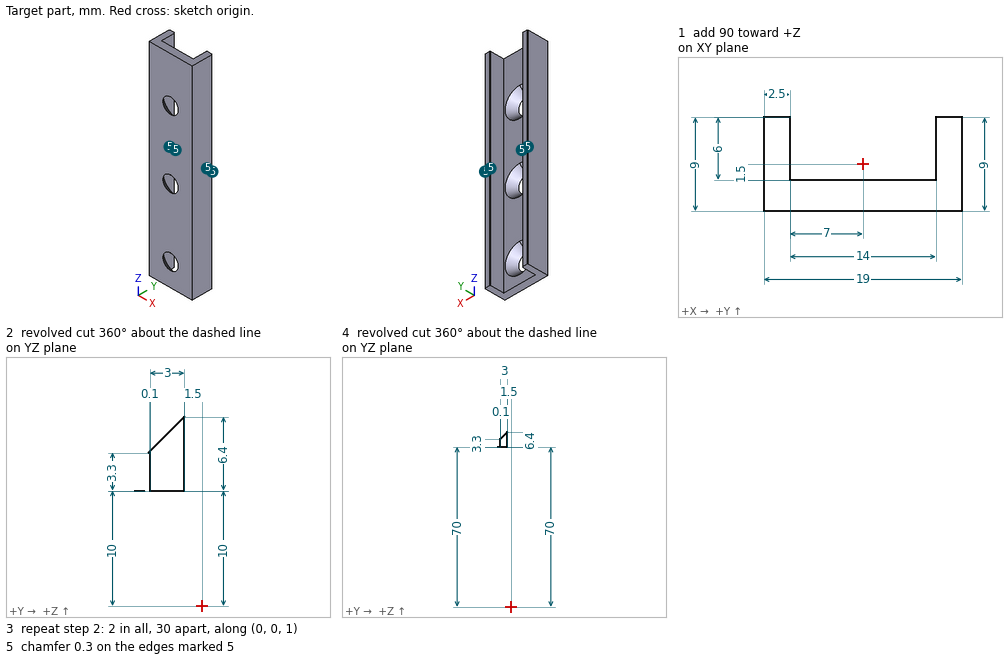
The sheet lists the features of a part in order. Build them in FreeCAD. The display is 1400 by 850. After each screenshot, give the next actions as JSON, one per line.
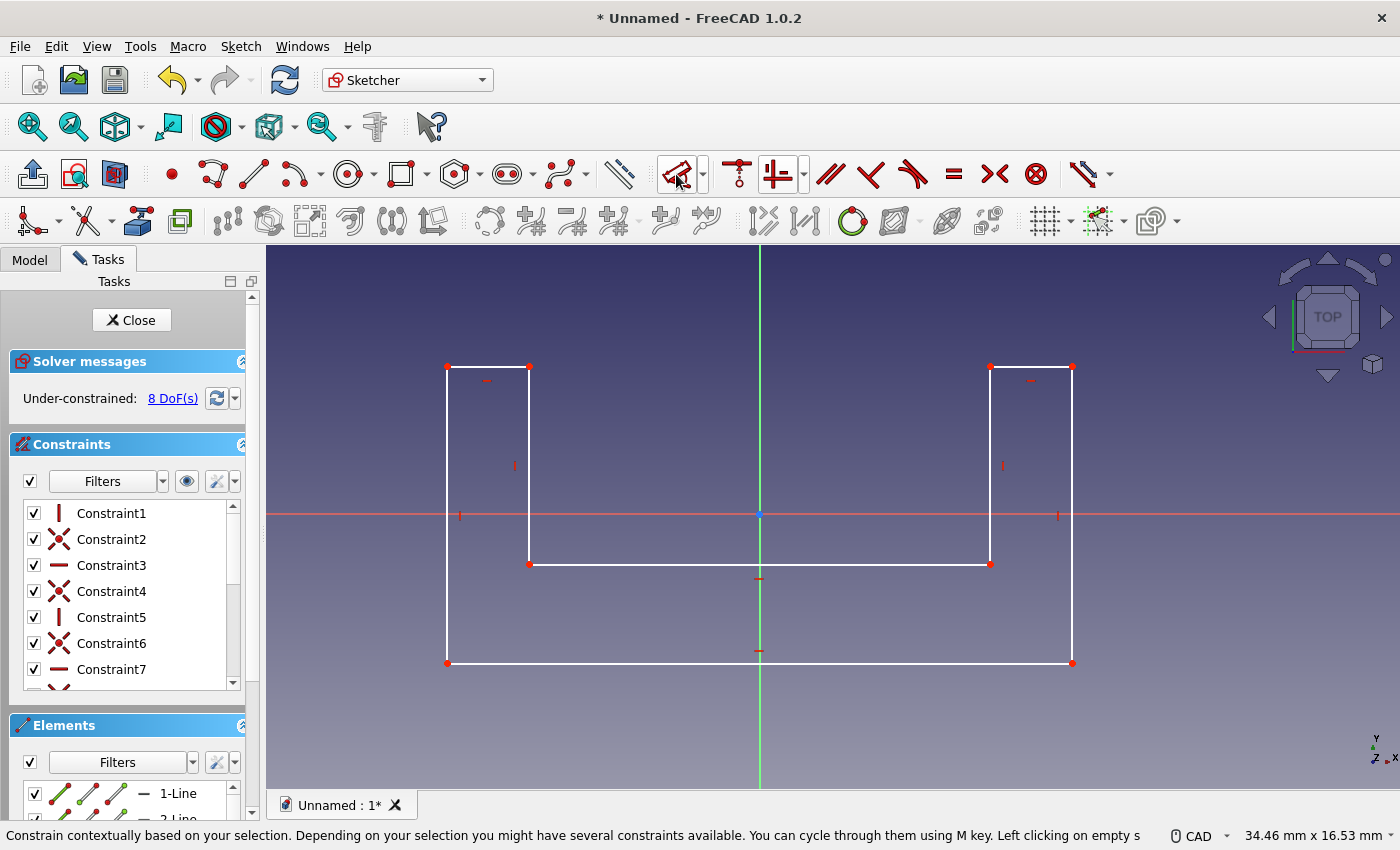
{"action": "left_click", "coordinate": [529, 426]}
{"action": "left_click", "coordinate": [495, 466]}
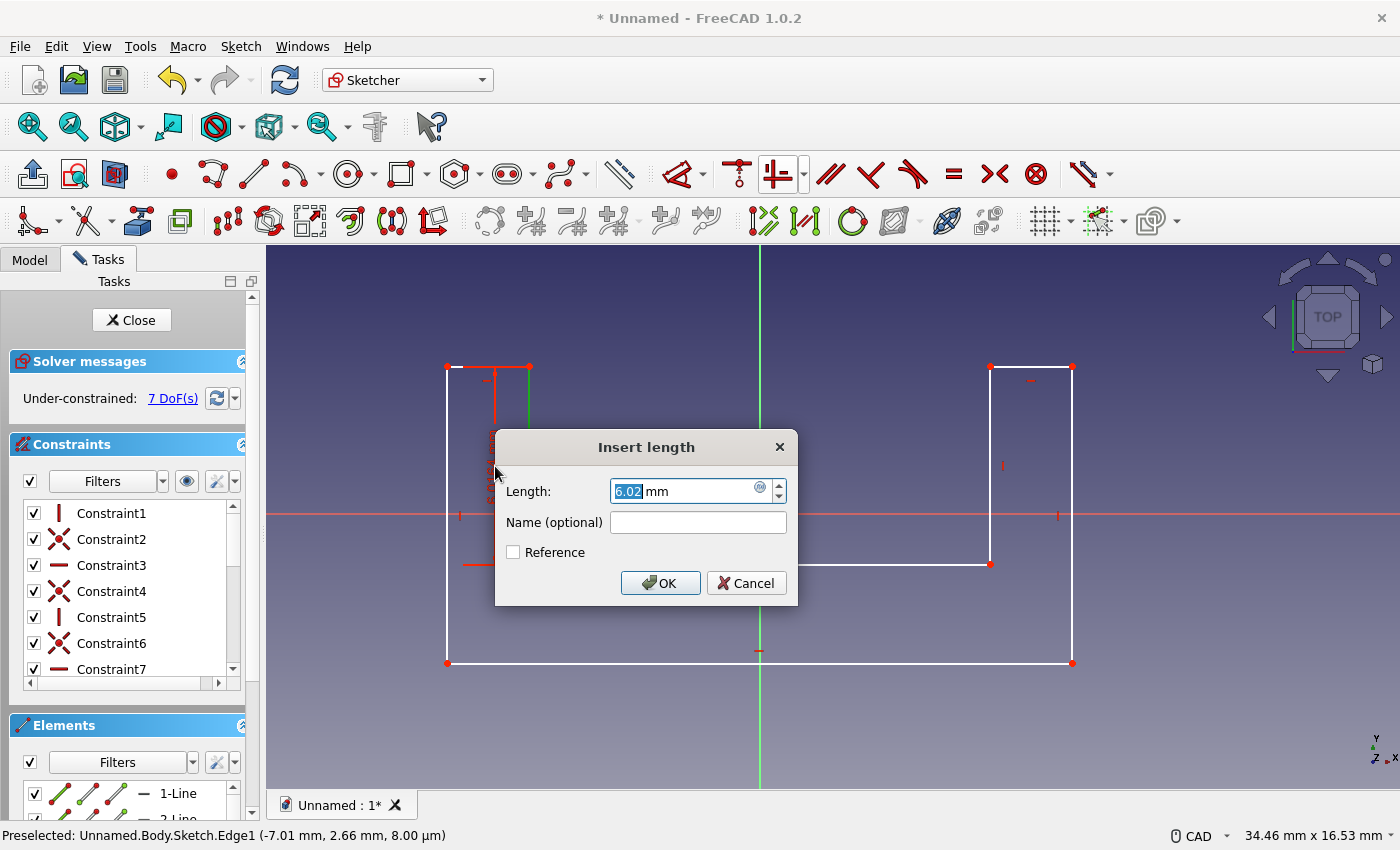
{"action": "type", "text": "6"}
{"action": "key", "text": "Return"}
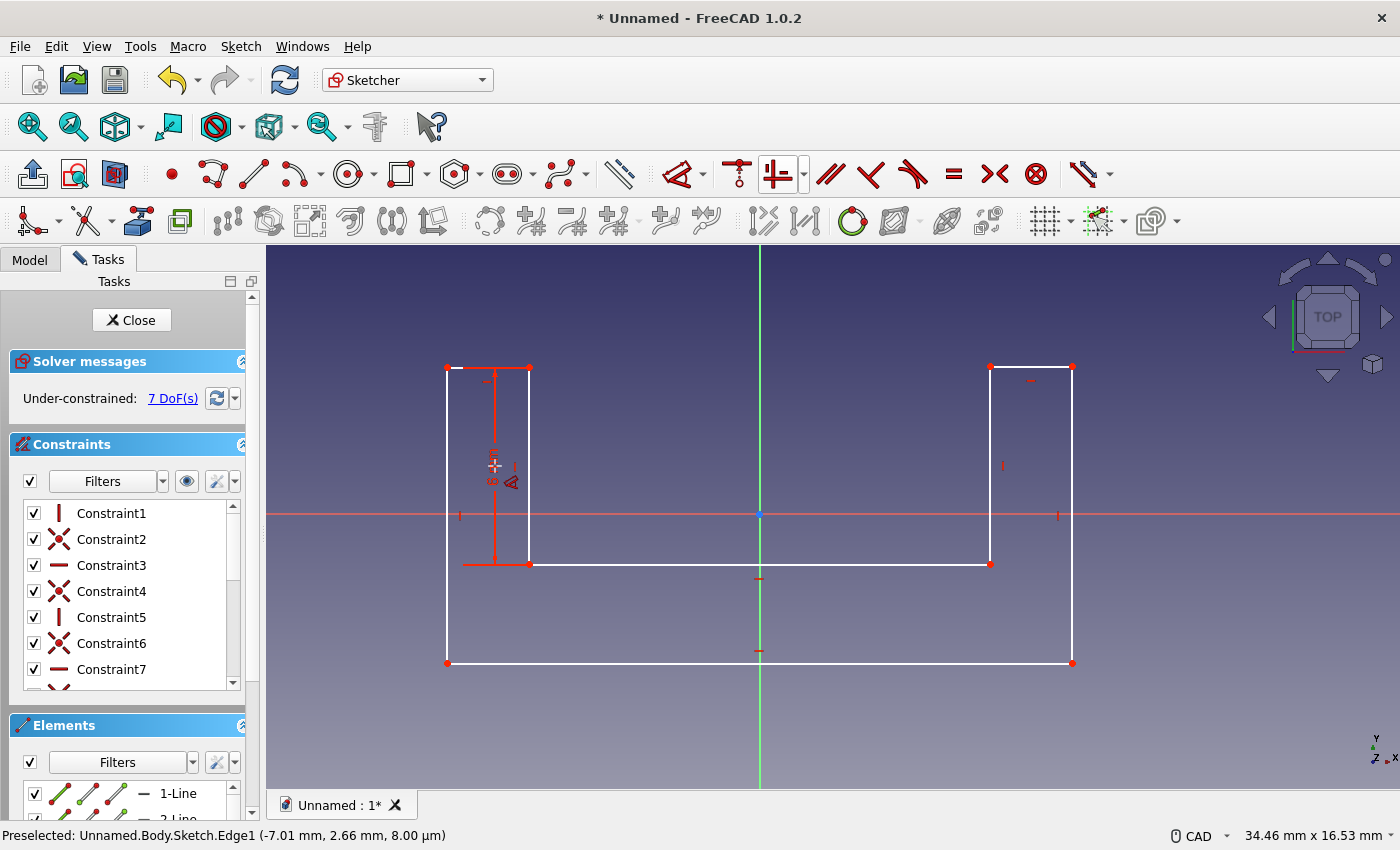
{"action": "left_click", "coordinate": [447, 456]}
{"action": "left_click", "coordinate": [413, 448]}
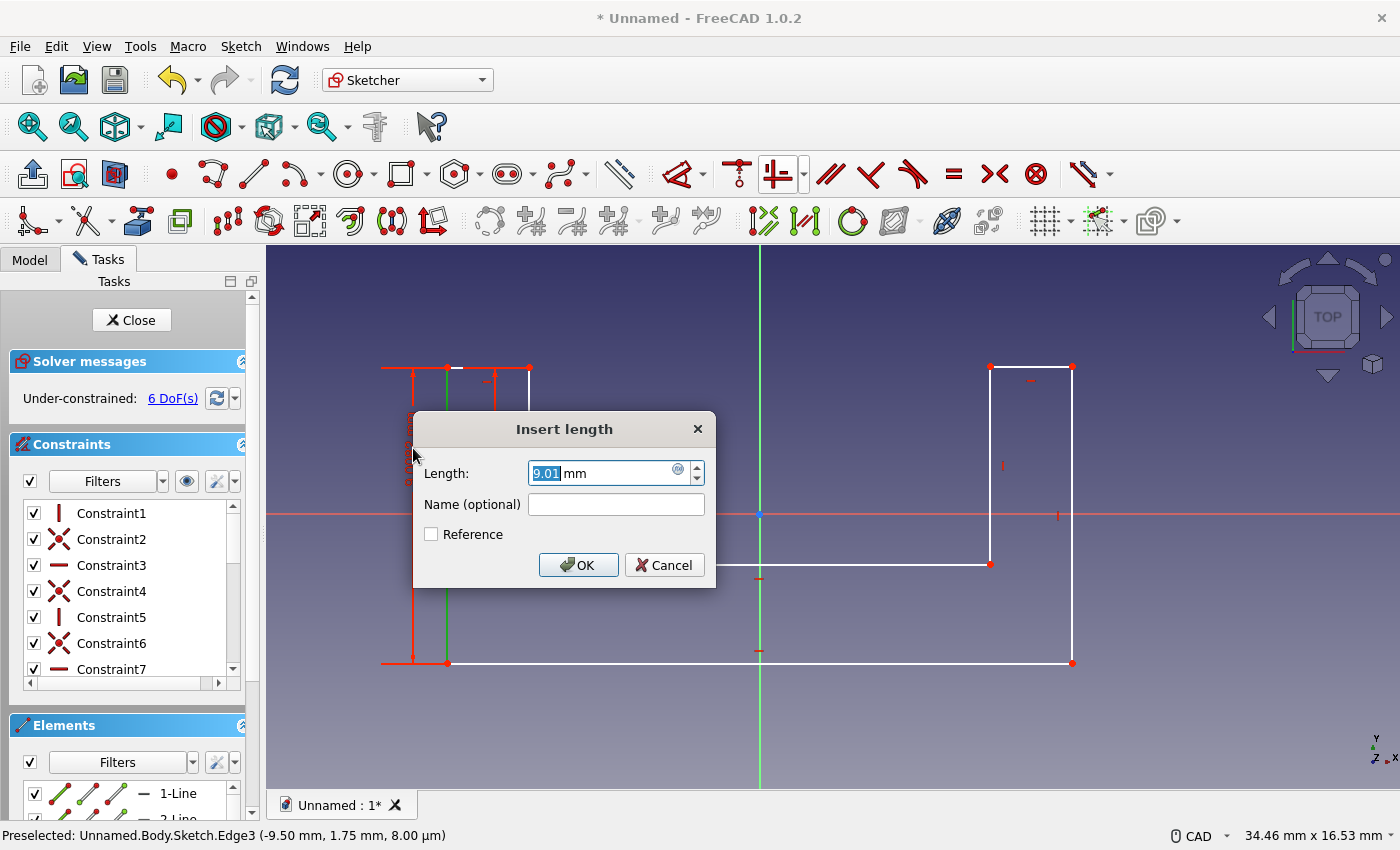
{"action": "type", "text": "9"}
{"action": "key", "text": "Return"}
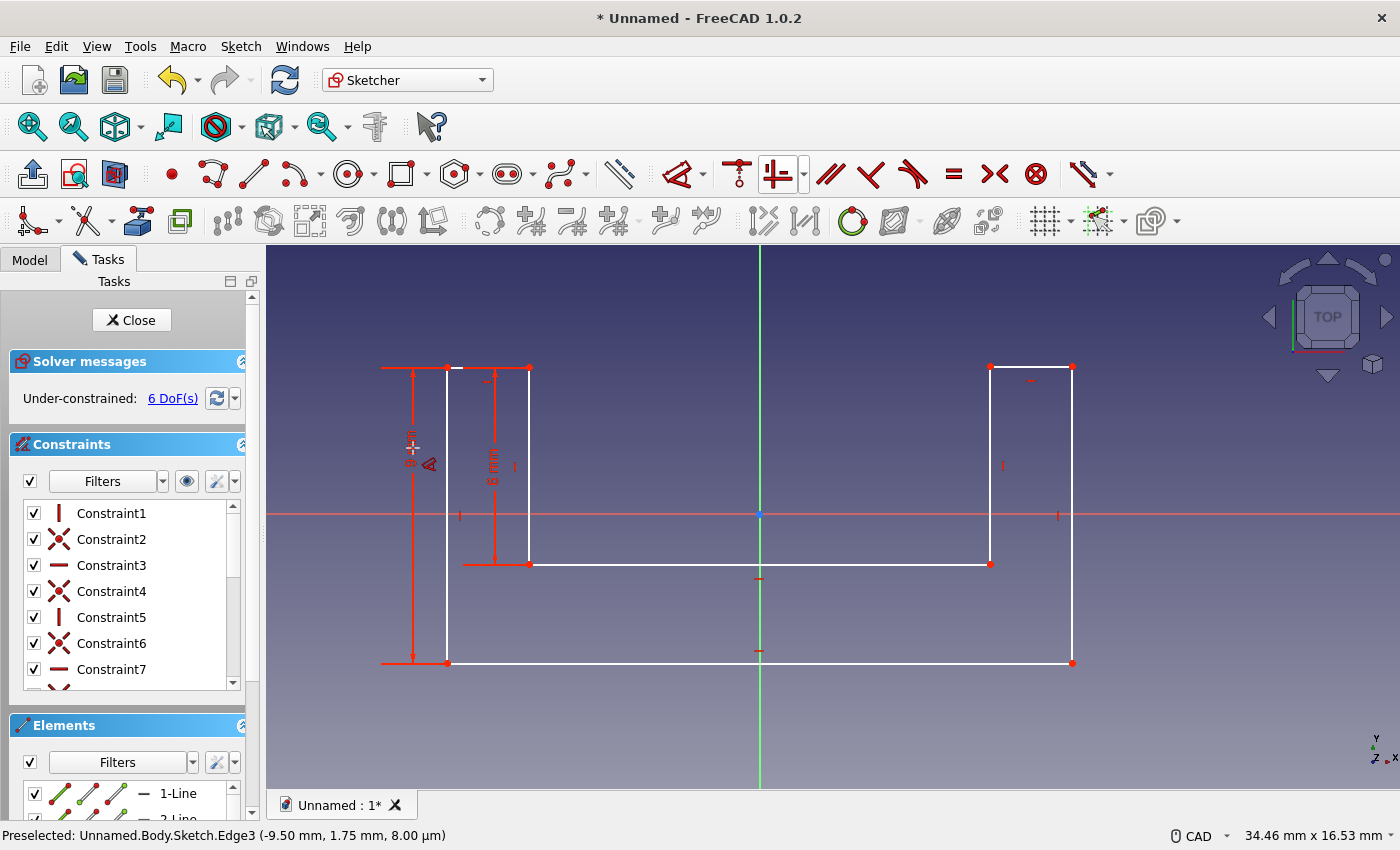
{"action": "left_click", "coordinate": [1072, 575]}
{"action": "left_click", "coordinate": [1106, 447]}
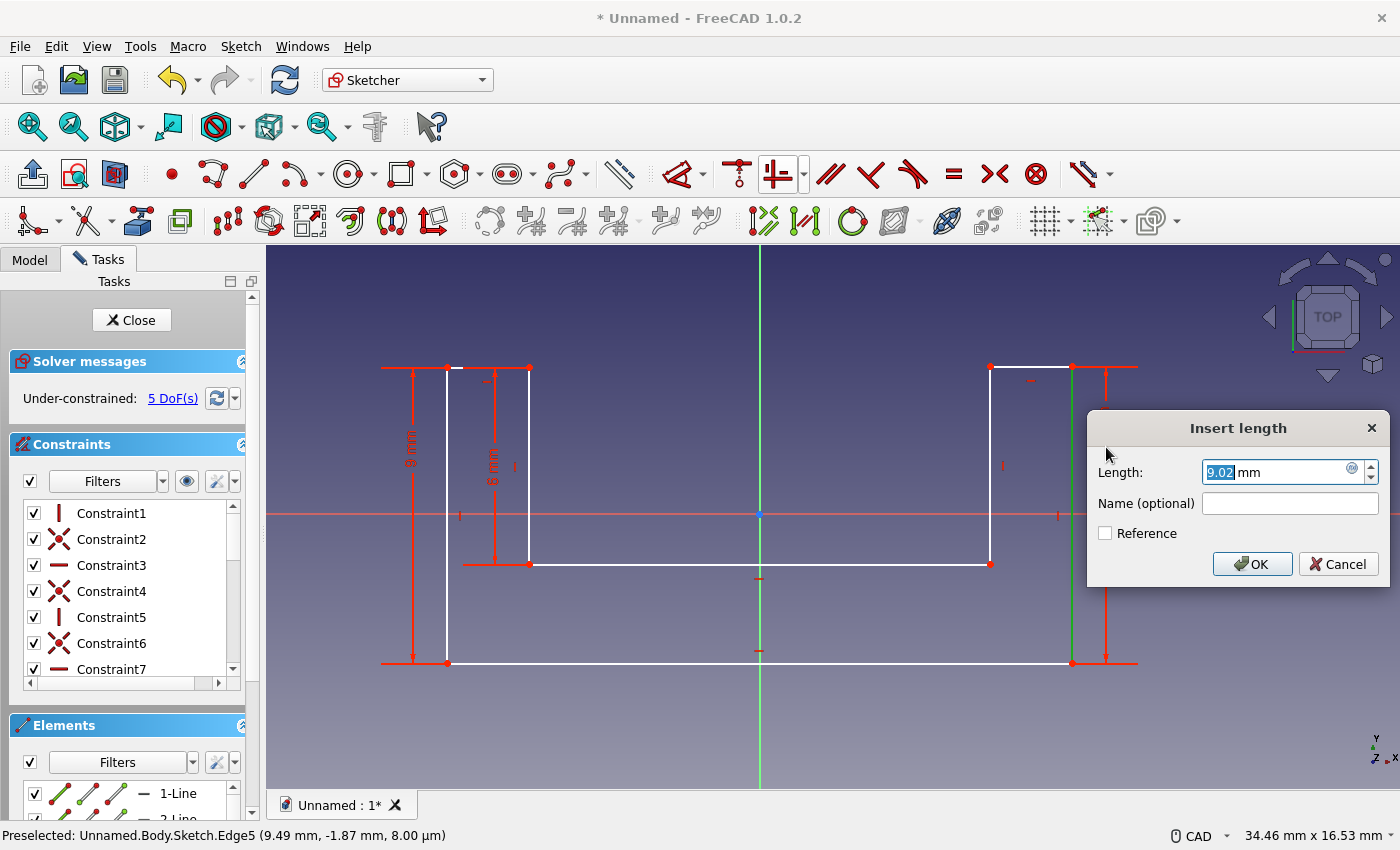
{"action": "type", "text": "9"}
{"action": "key", "text": "Return"}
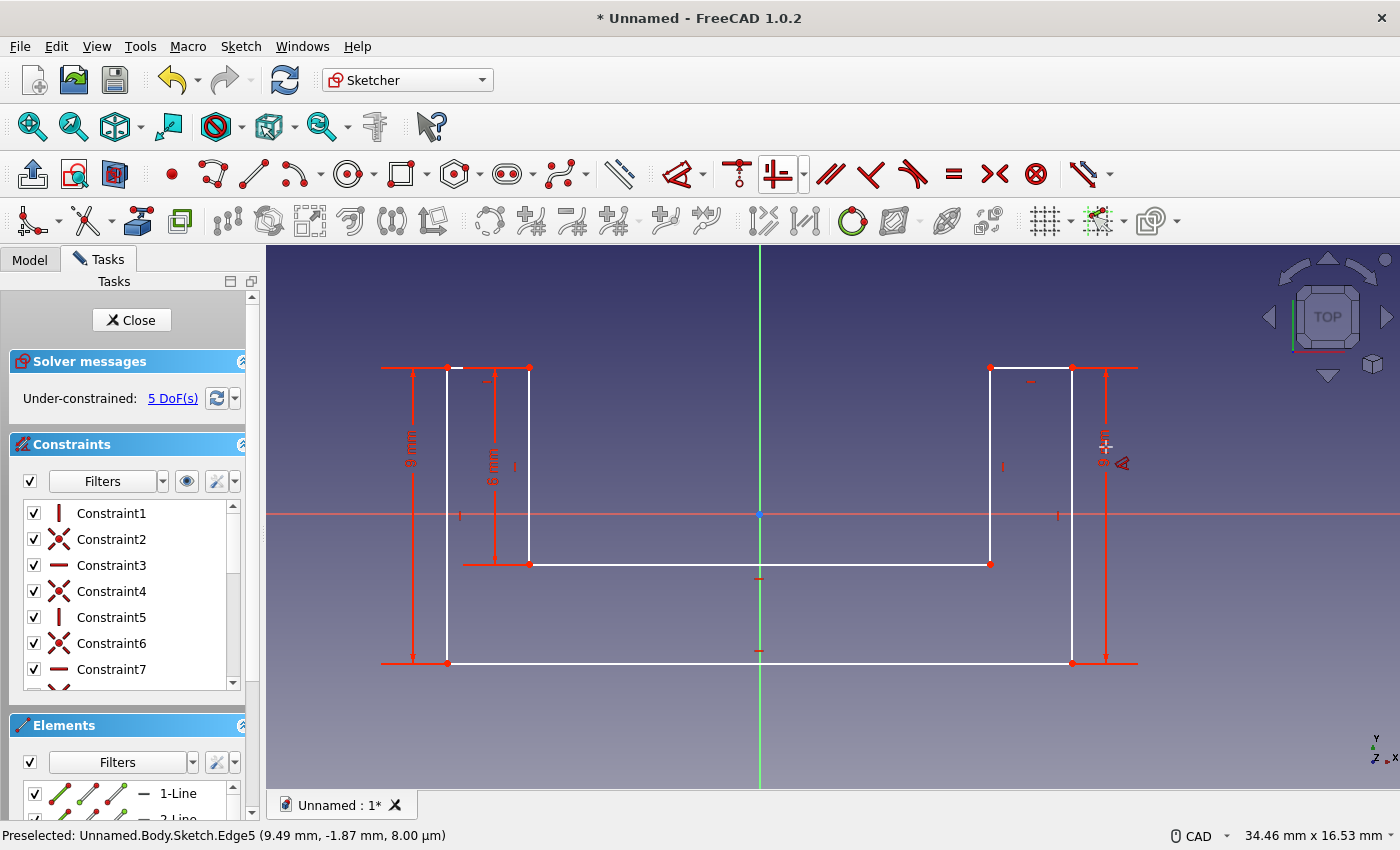
{"action": "left_click", "coordinate": [635, 664]}
{"action": "left_click", "coordinate": [616, 698]}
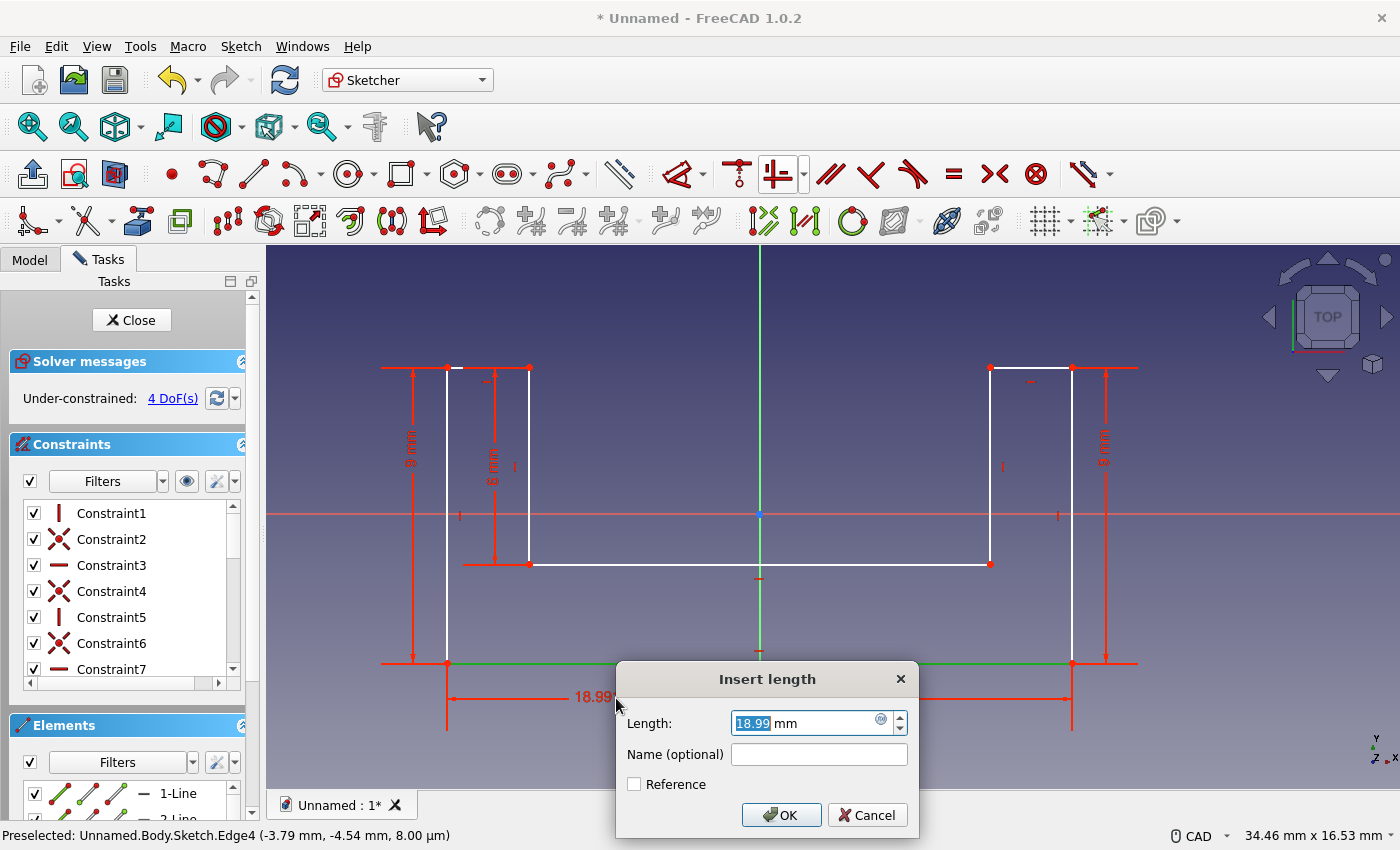
{"action": "type", "text": "19"}
{"action": "key", "text": "Return"}